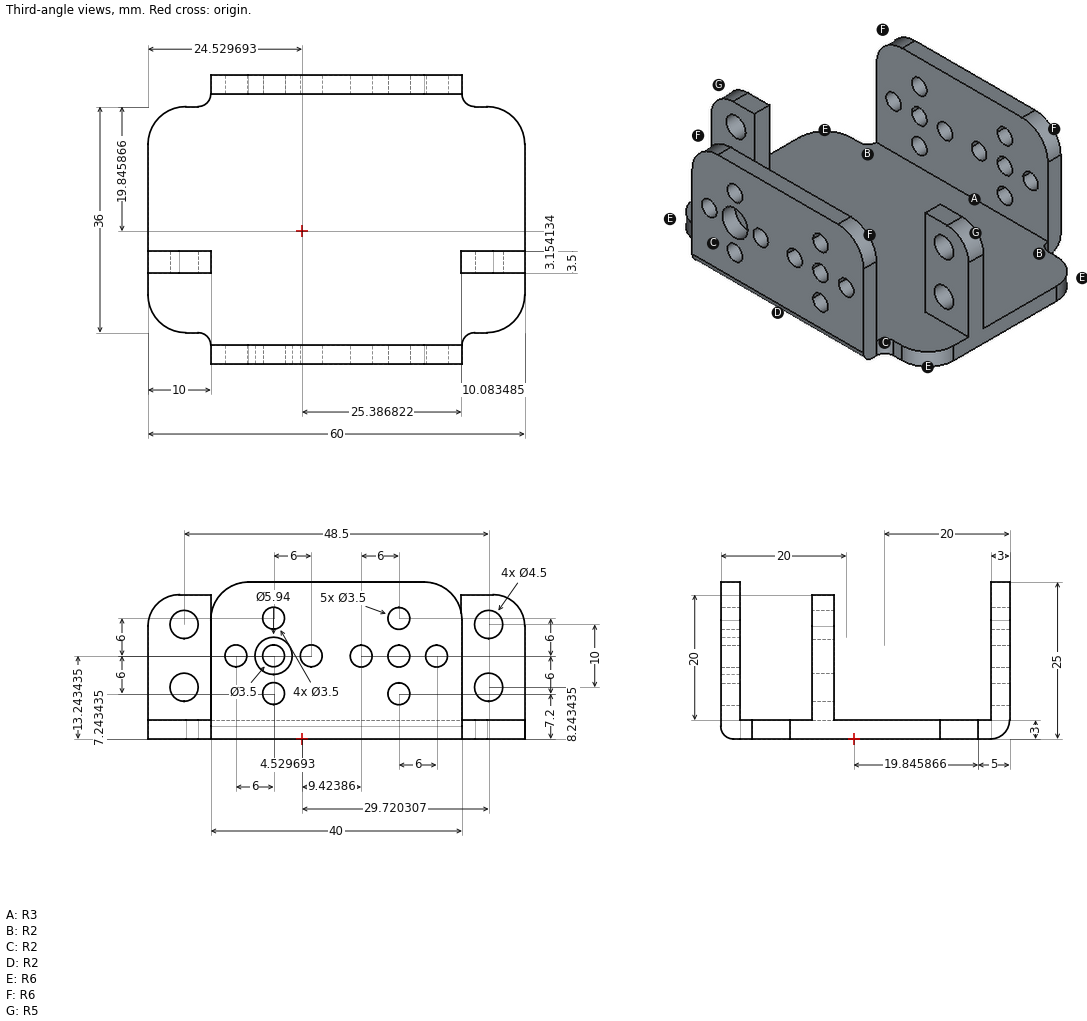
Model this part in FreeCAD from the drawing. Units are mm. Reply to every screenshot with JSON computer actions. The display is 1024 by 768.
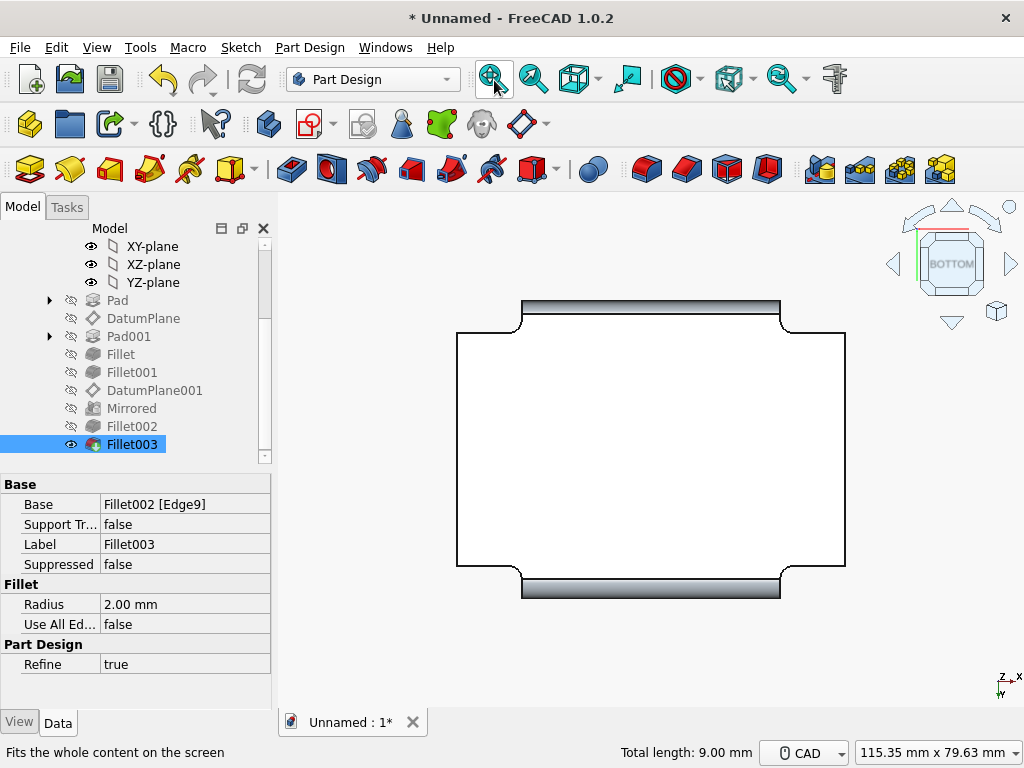
{"action": "key", "text": "4"}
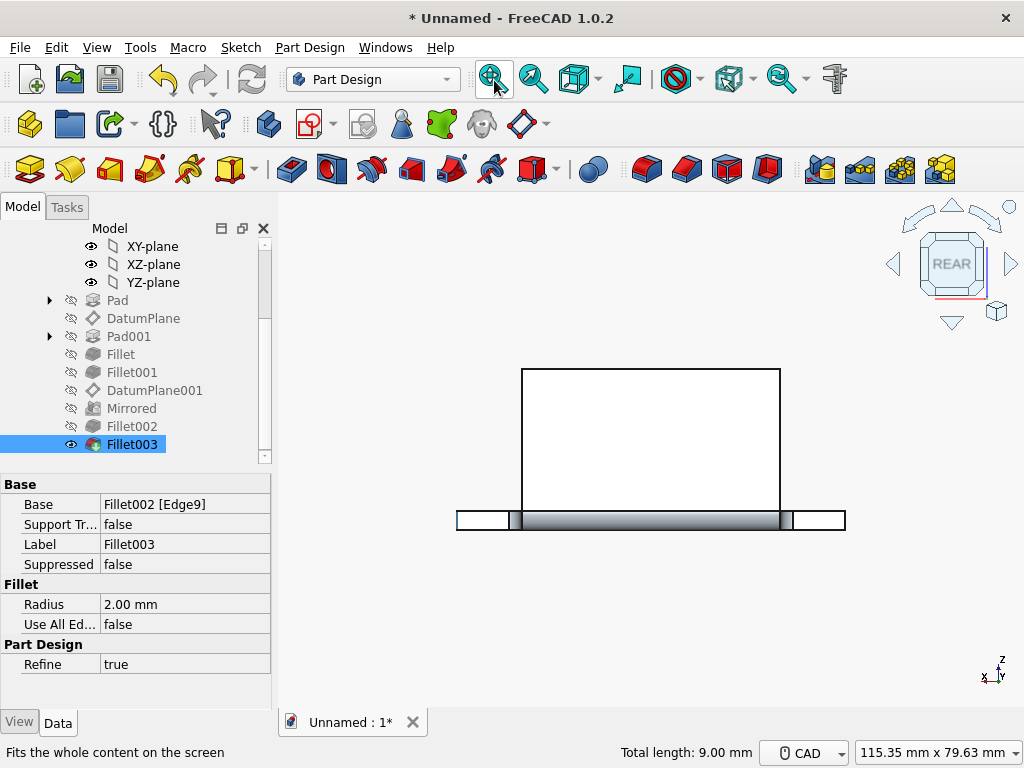
{"action": "left_click", "coordinate": [845, 520], "text": "ctrl"}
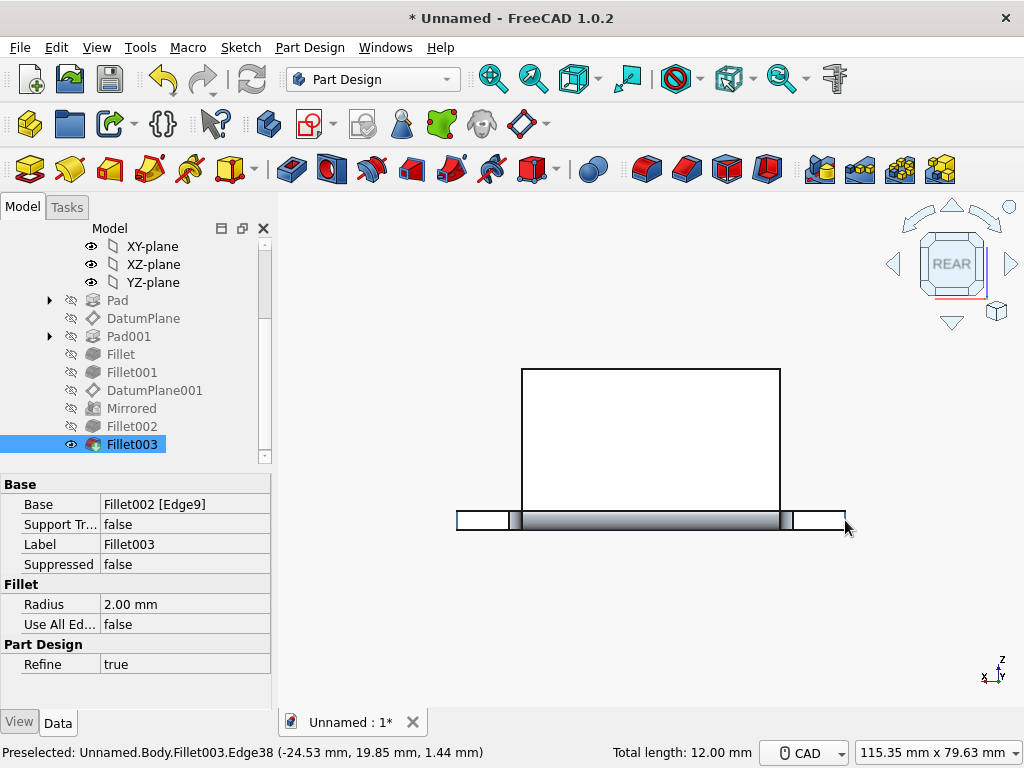
{"action": "left_click", "coordinate": [648, 170]}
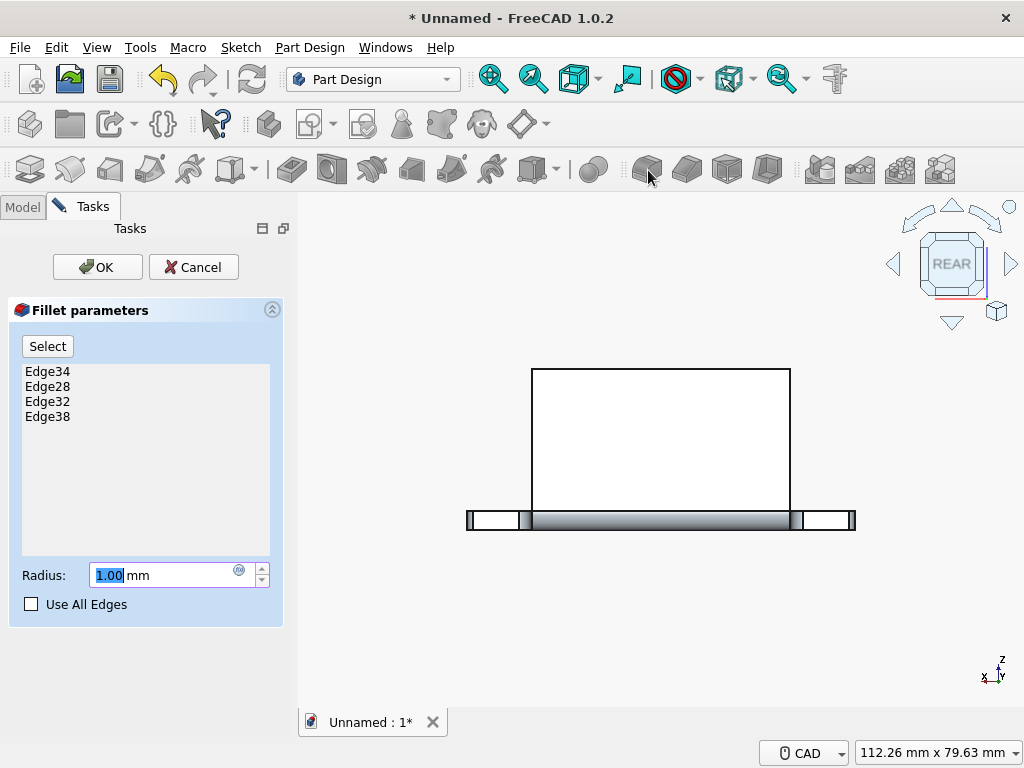
{"action": "type", "text": "6"}
{"action": "key", "text": "Tab"}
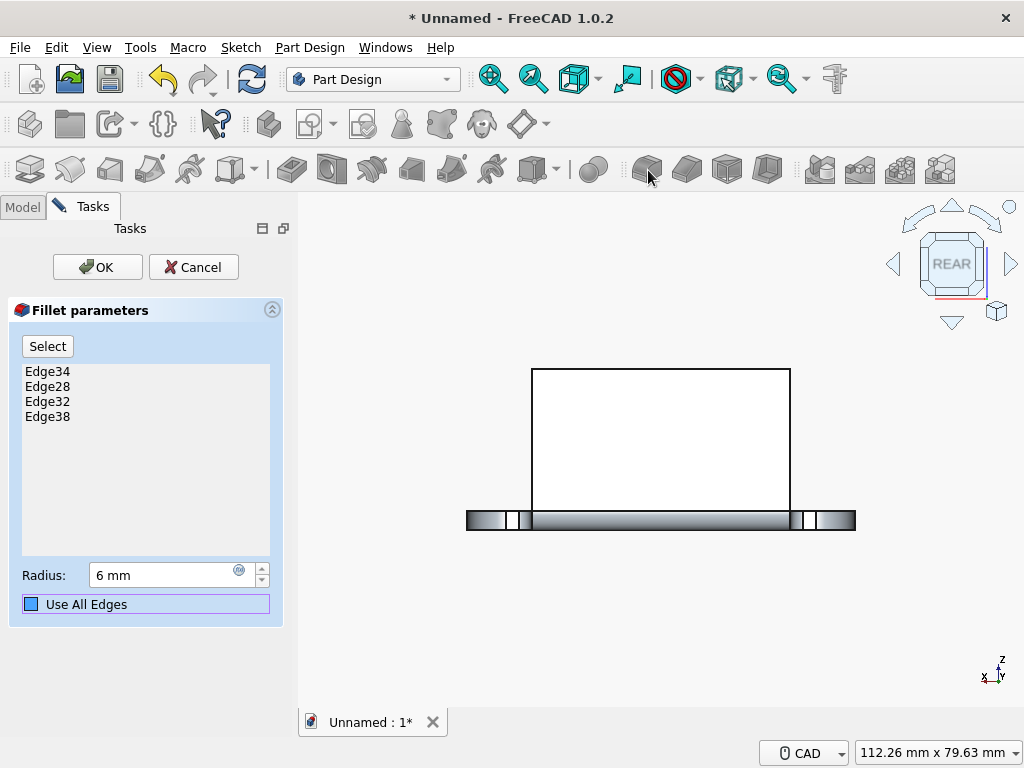
{"action": "left_click", "coordinate": [98, 267]}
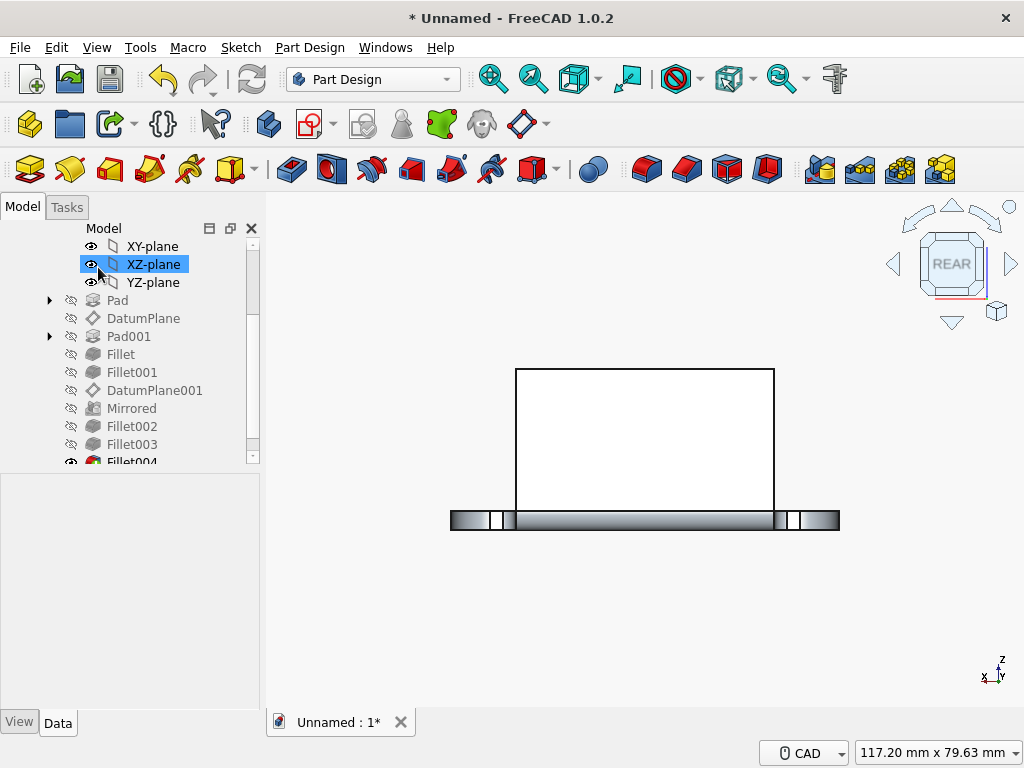
{"action": "scroll", "coordinate": [774, 368], "scroll_direction": "up", "scroll_amount": 4}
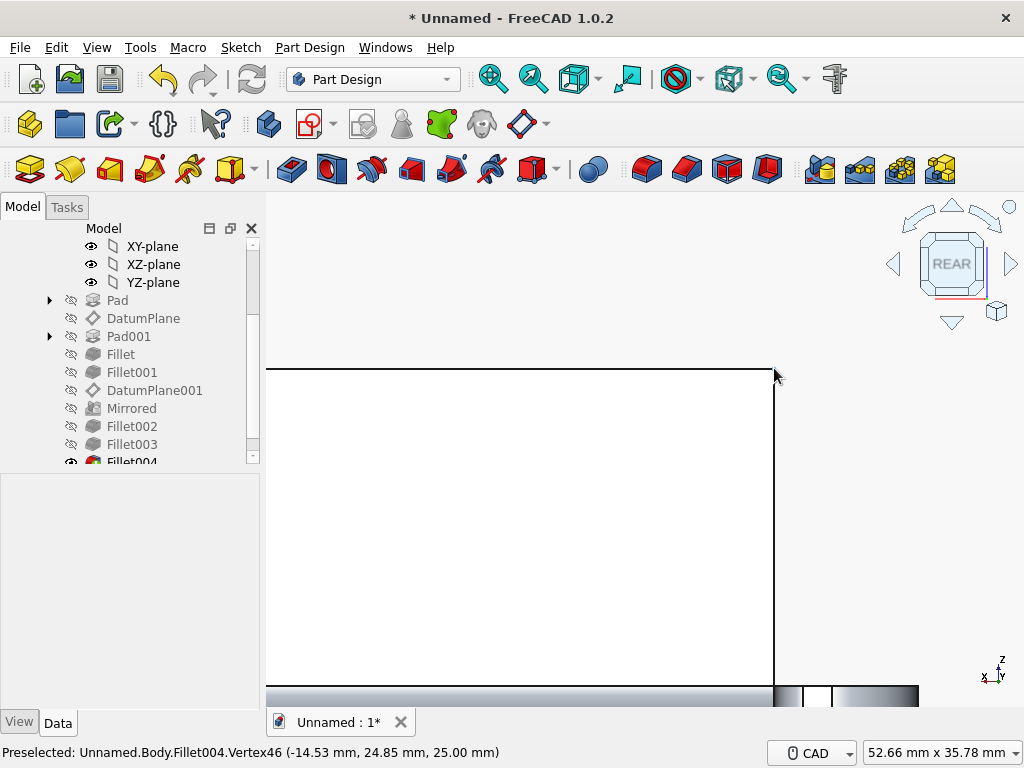
{"action": "left_click", "coordinate": [494, 80]}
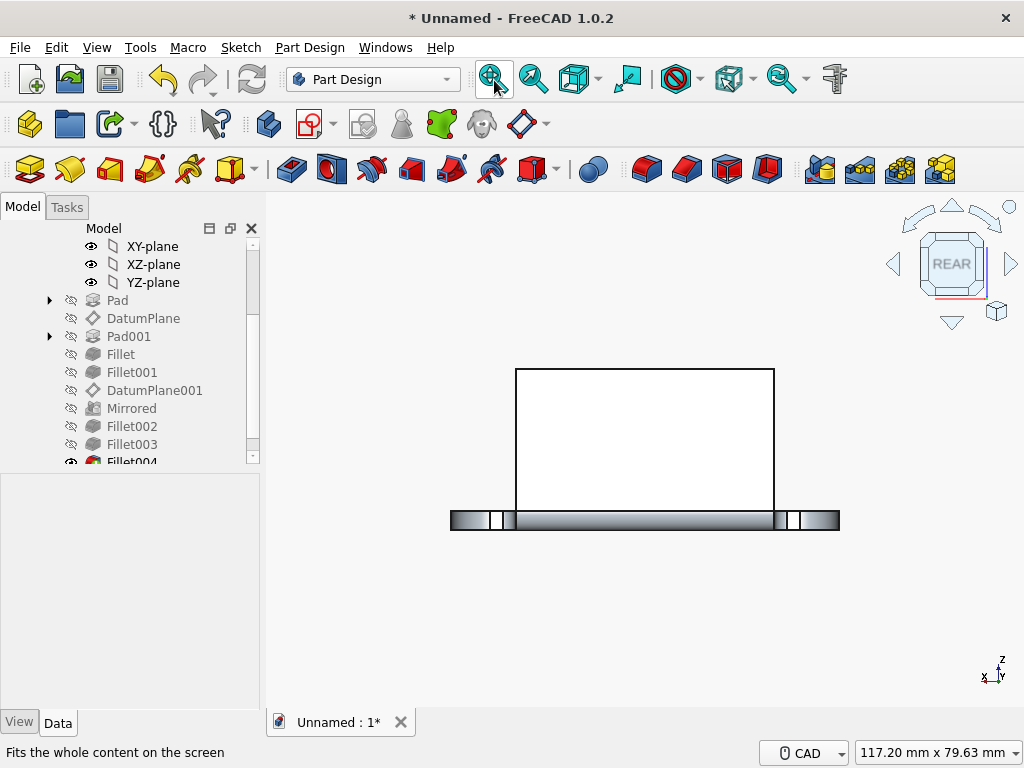
{"action": "key", "text": "0"}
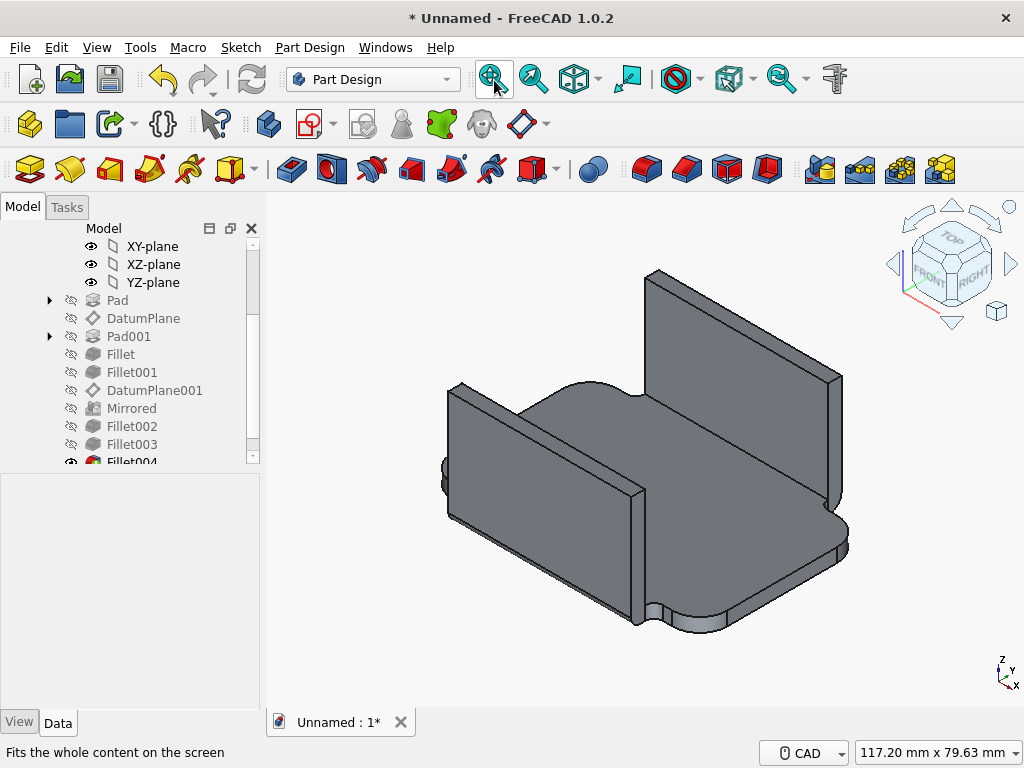
{"action": "left_click", "coordinate": [835, 379]}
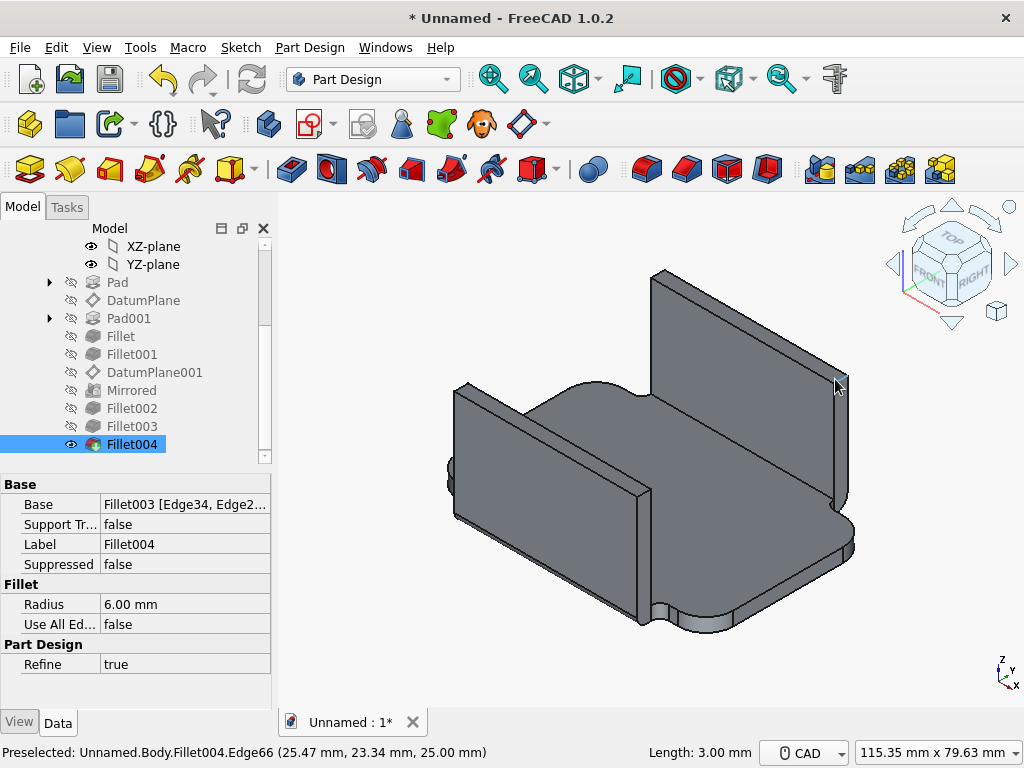
{"action": "left_click", "coordinate": [644, 492], "text": "ctrl"}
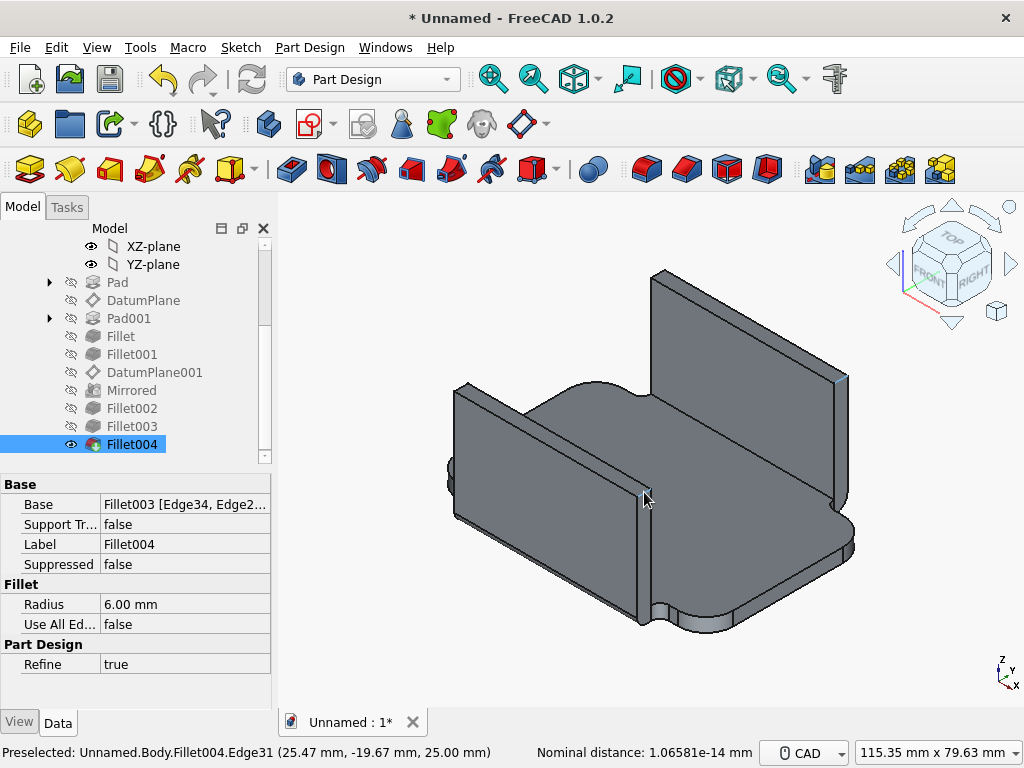
{"action": "scroll", "coordinate": [658, 273], "scroll_direction": "up", "scroll_amount": 4}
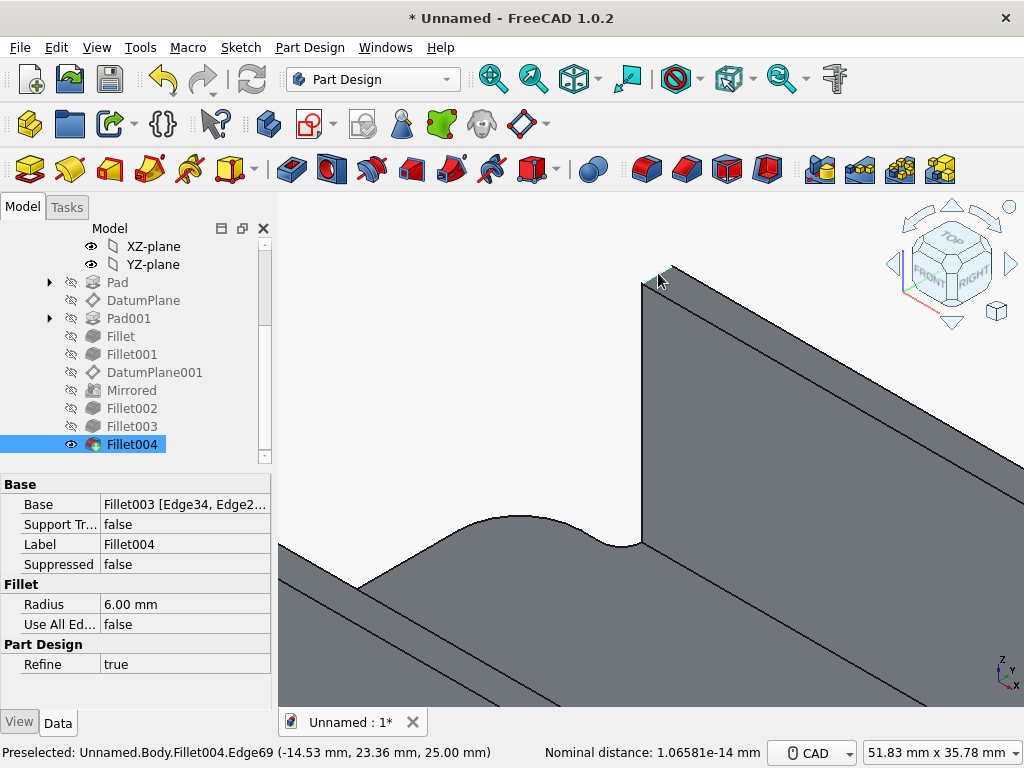
{"action": "left_click", "coordinate": [494, 80]}